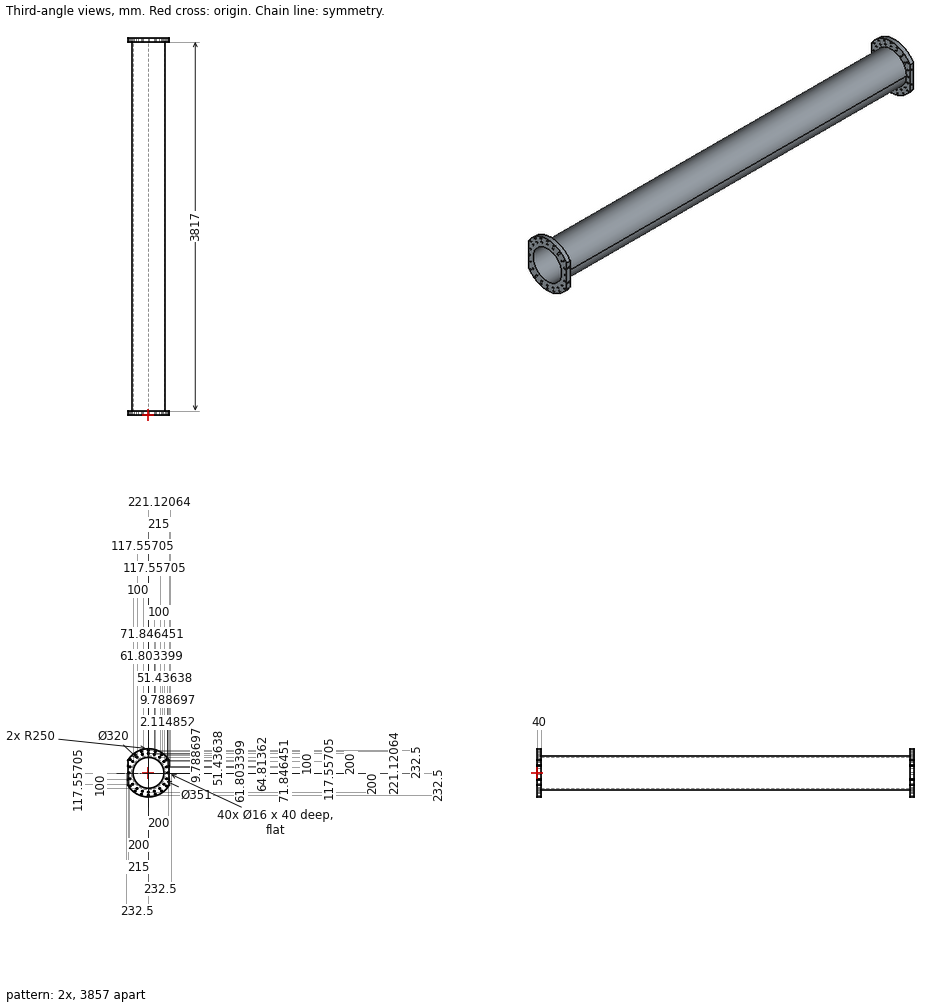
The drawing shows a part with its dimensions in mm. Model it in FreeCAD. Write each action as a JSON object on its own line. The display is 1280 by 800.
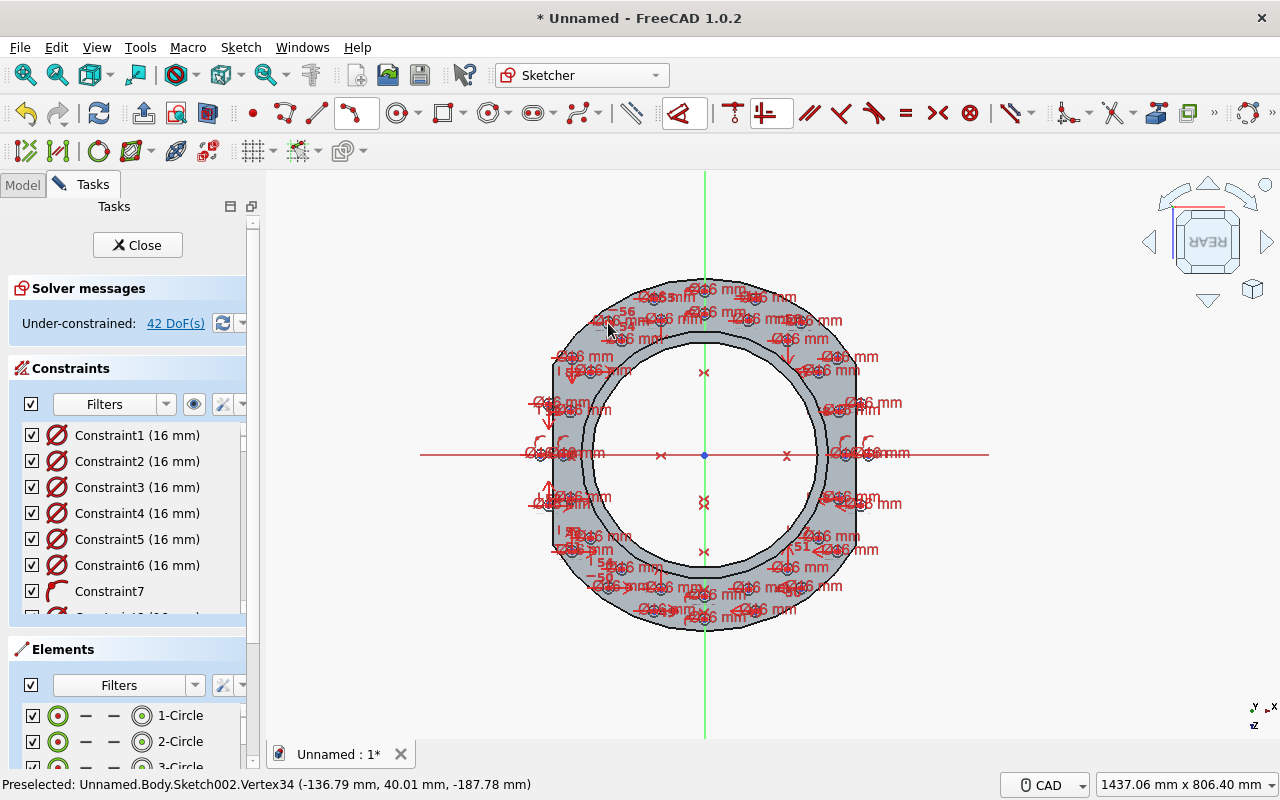
{"action": "left_click", "coordinate": [470, 455]}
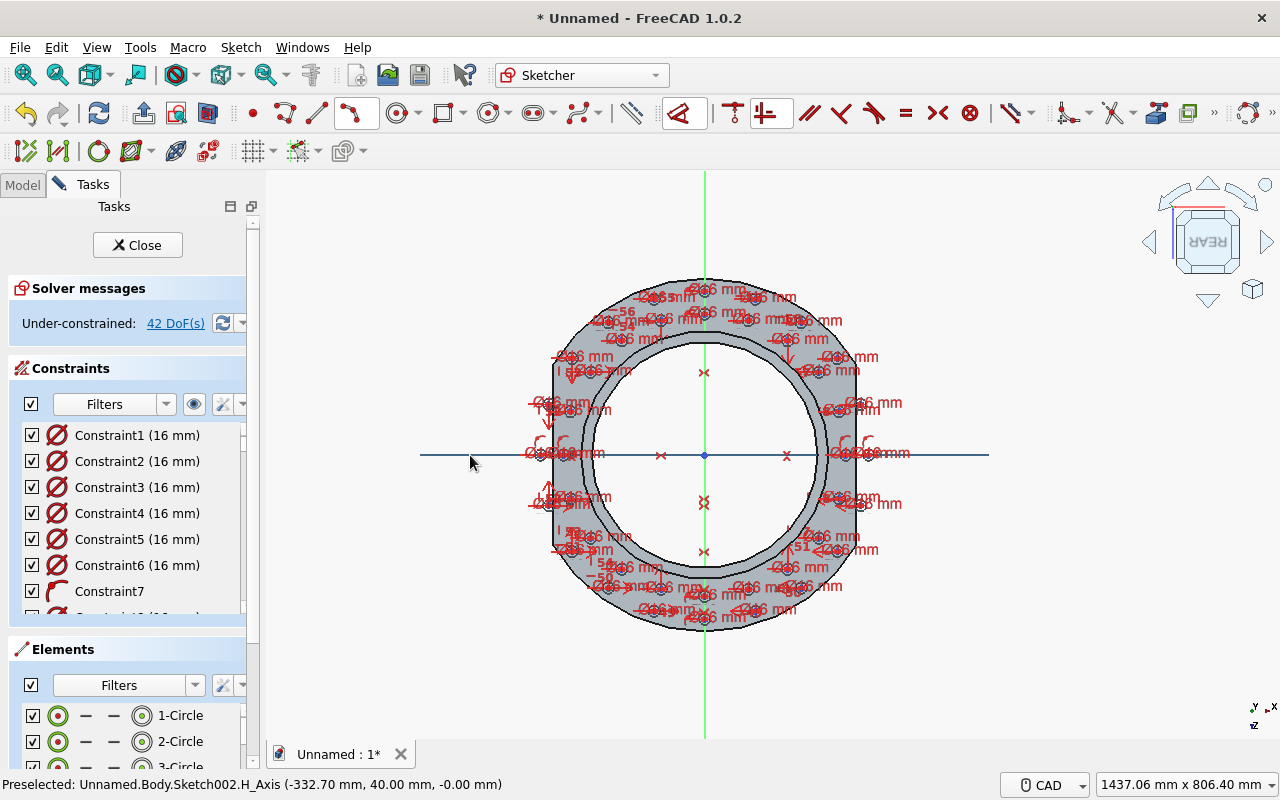
{"action": "key", "text": "s"}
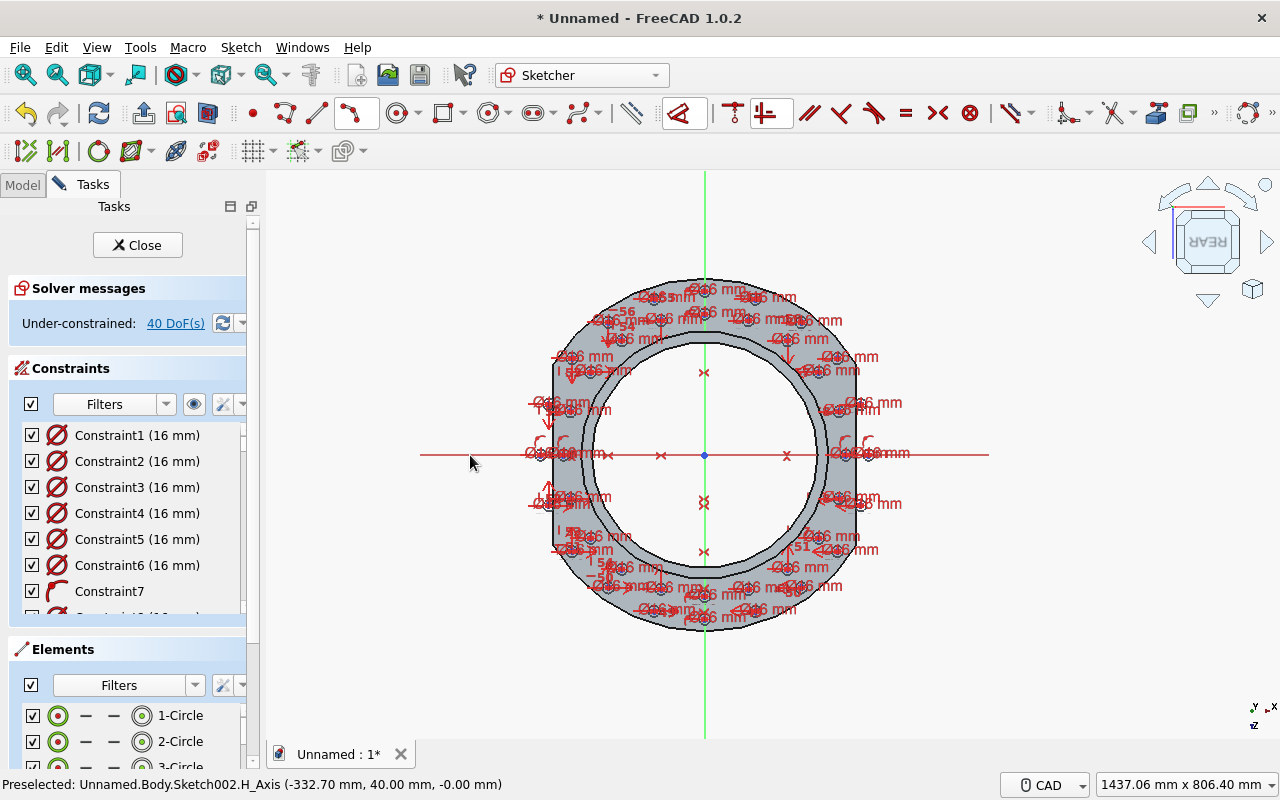
{"action": "scroll", "coordinate": [654, 611], "scroll_direction": "up", "scroll_amount": 4}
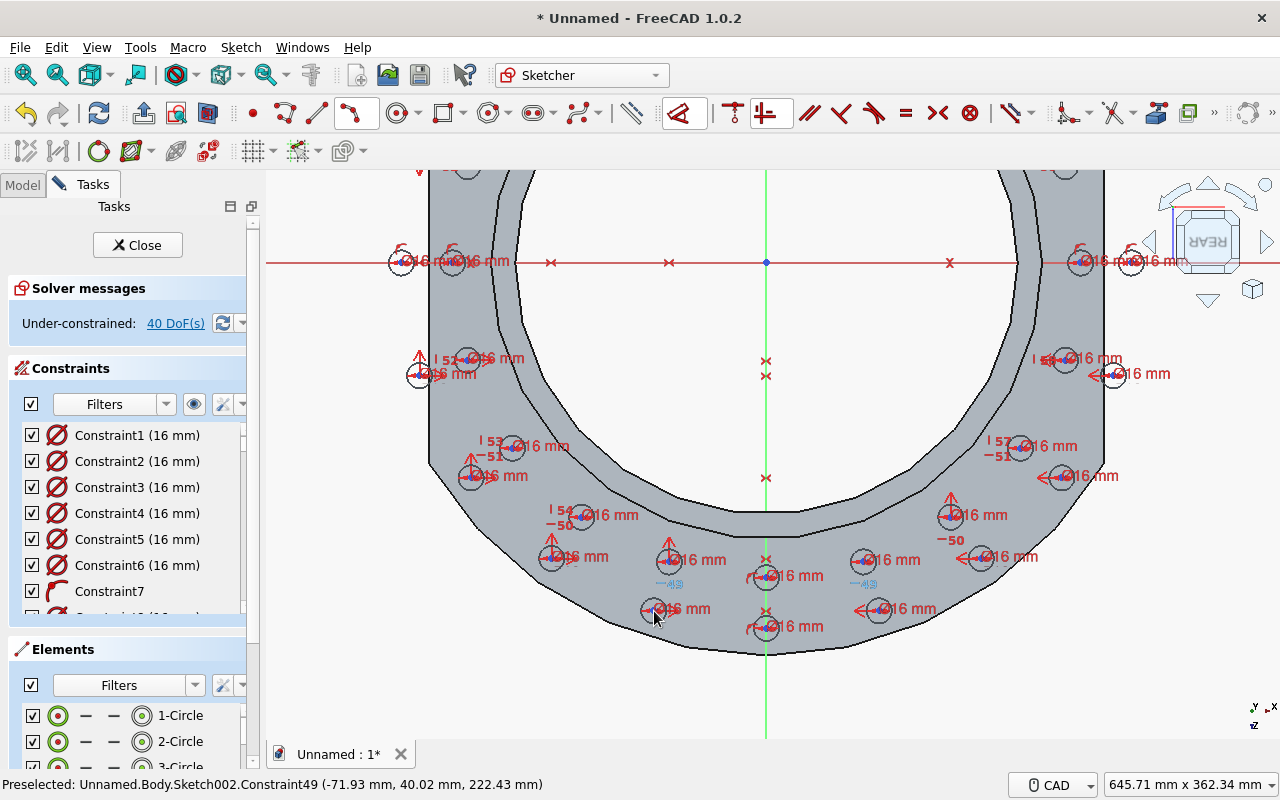
{"action": "left_click", "coordinate": [654, 611]}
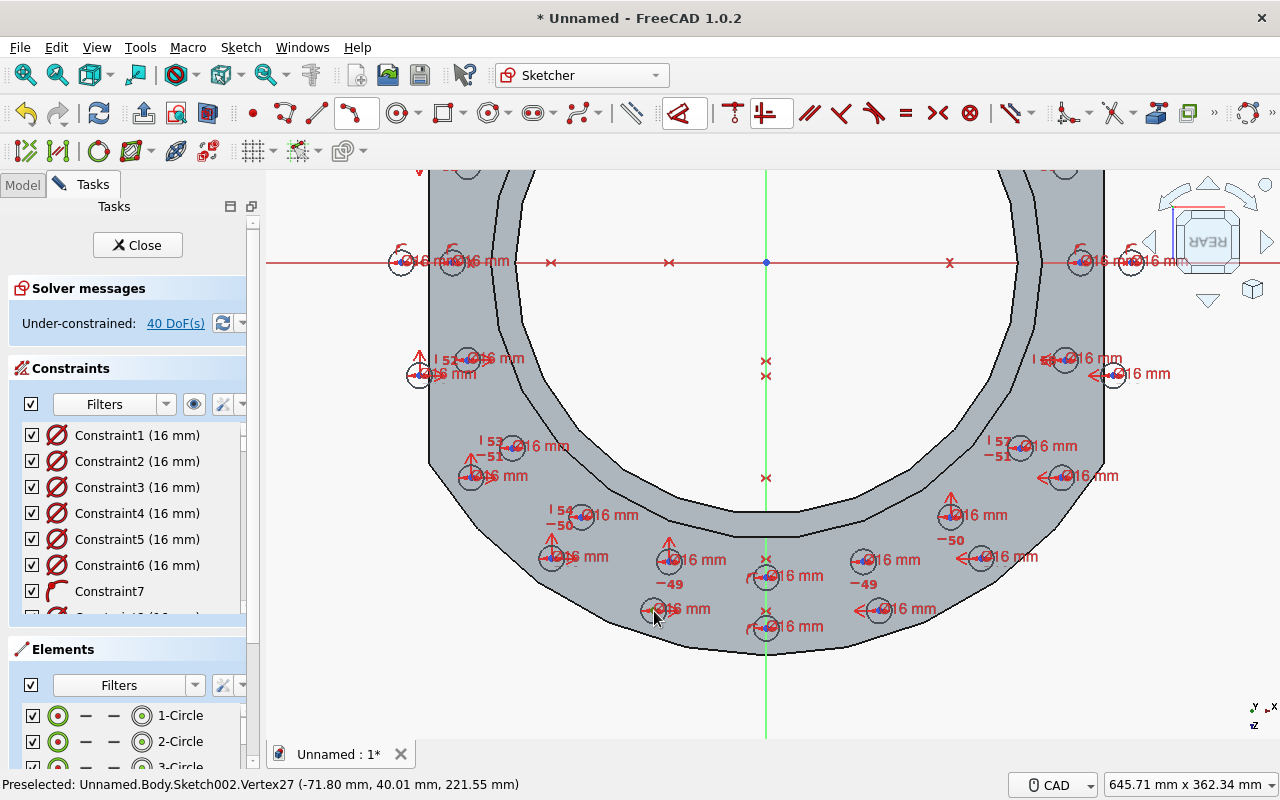
{"action": "scroll", "coordinate": [654, 611], "scroll_direction": "down", "scroll_amount": 4}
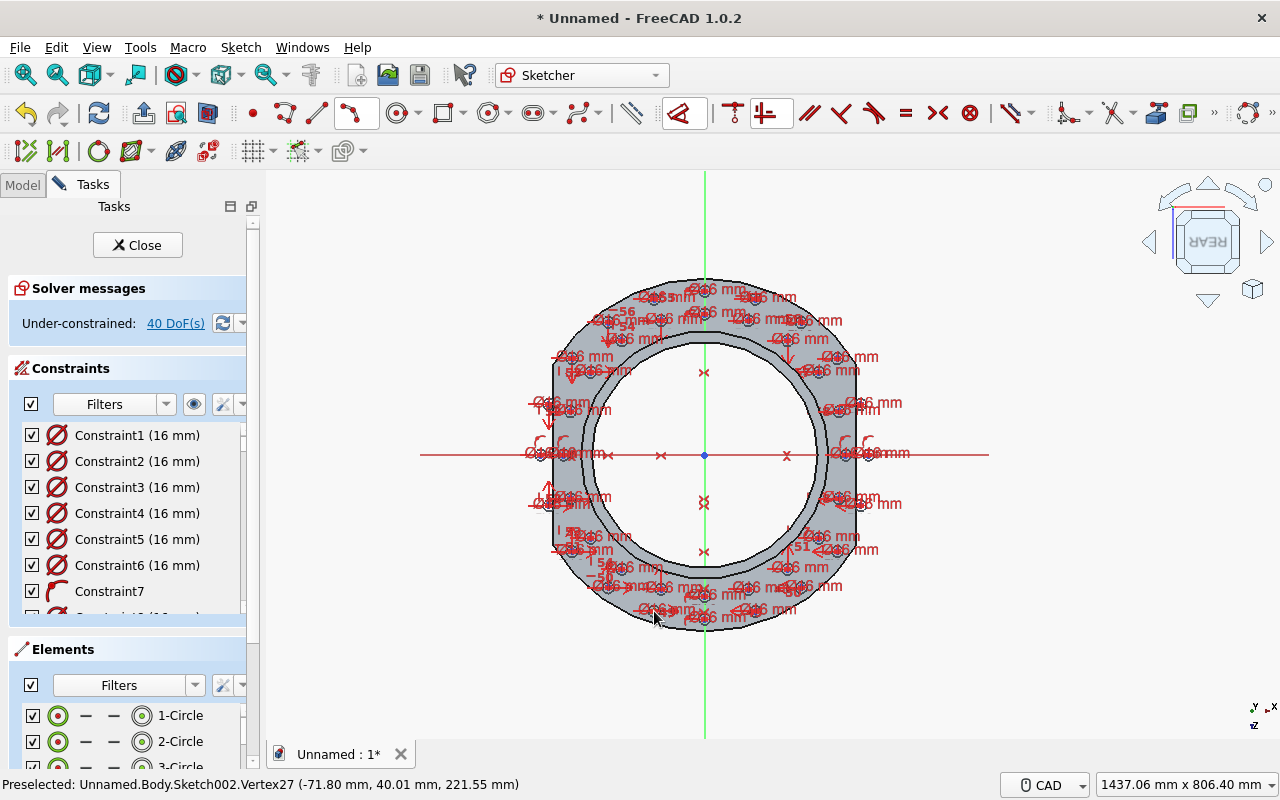
{"action": "left_click", "coordinate": [654, 299]}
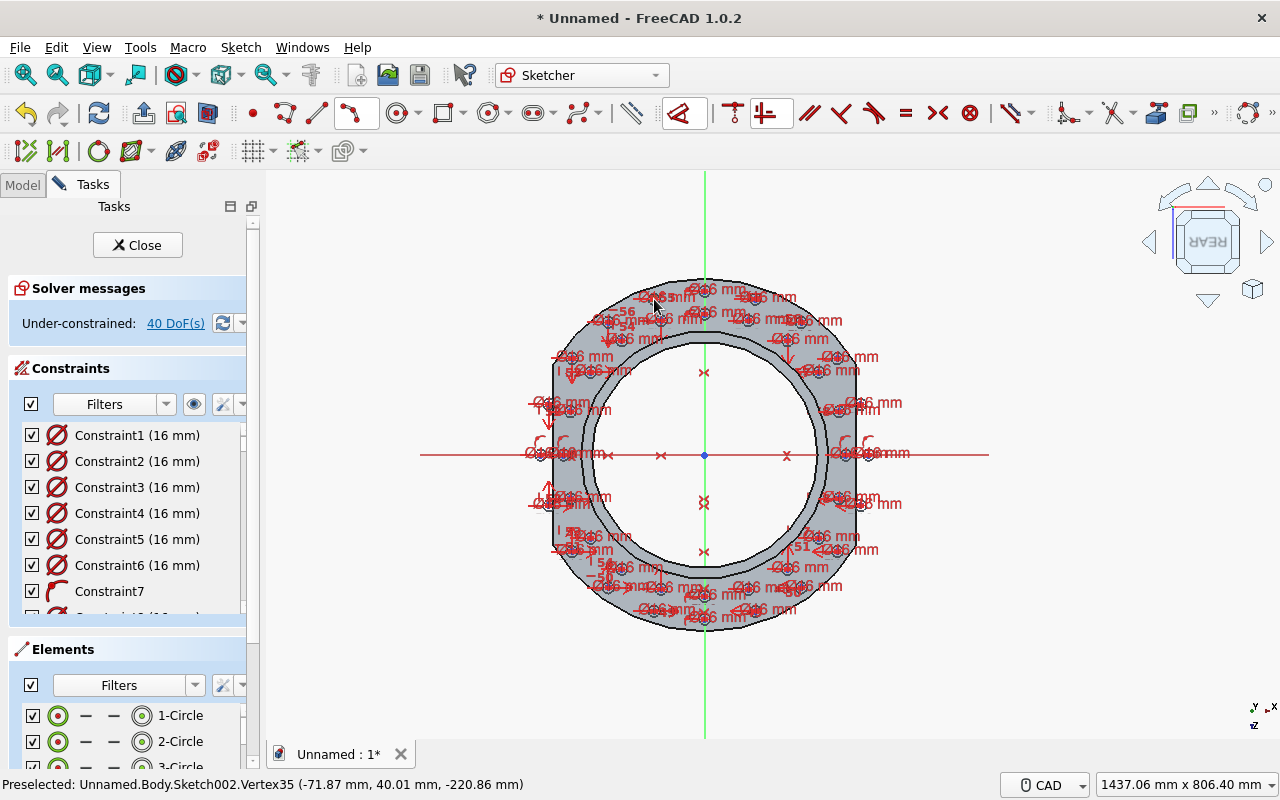
{"action": "left_click", "coordinate": [470, 455]}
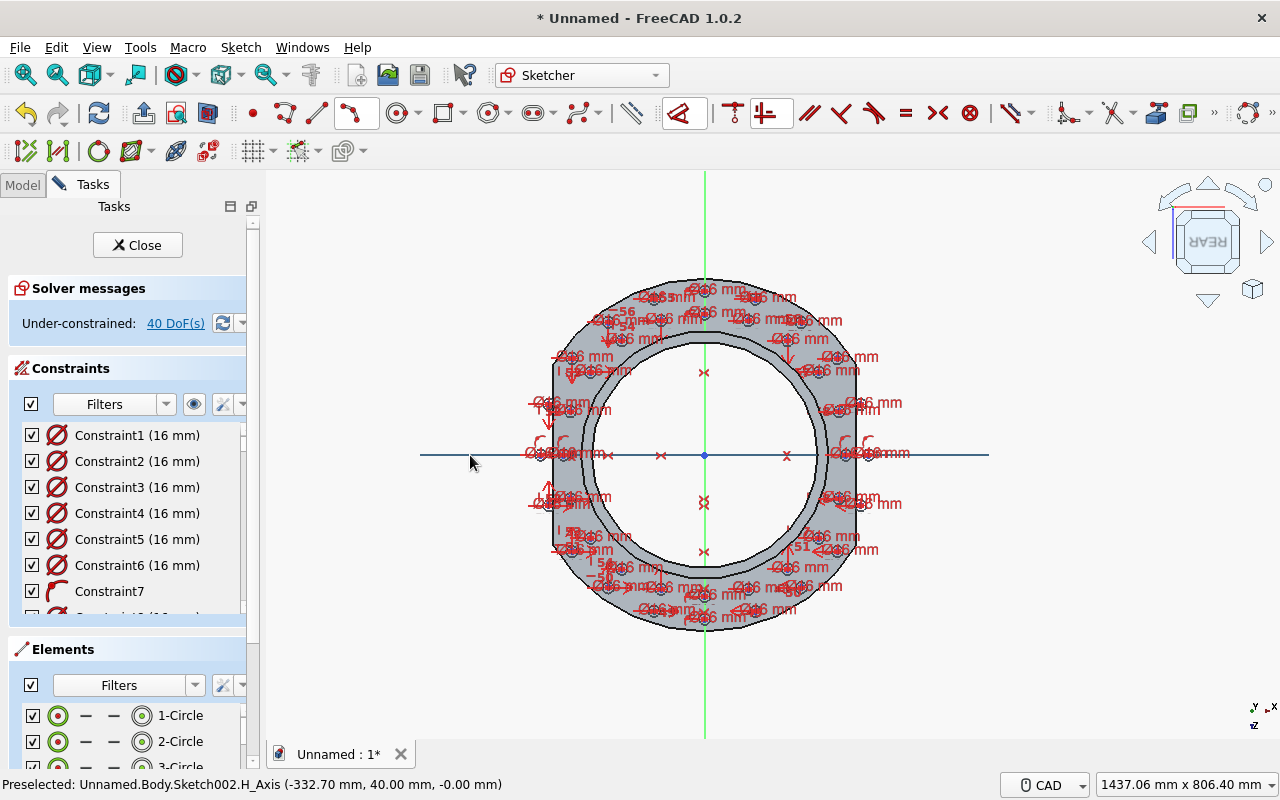
{"action": "left_click", "coordinate": [938, 114]}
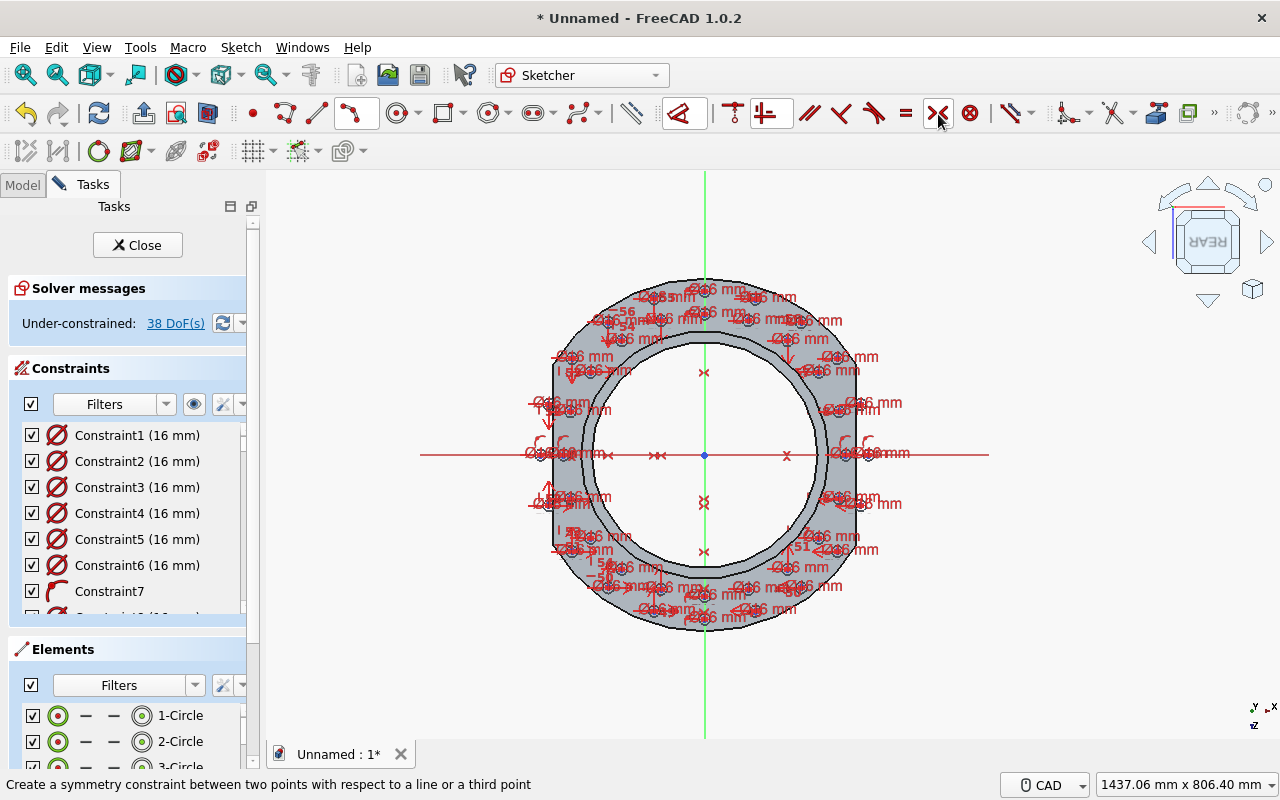
{"action": "left_click", "coordinate": [755, 611]}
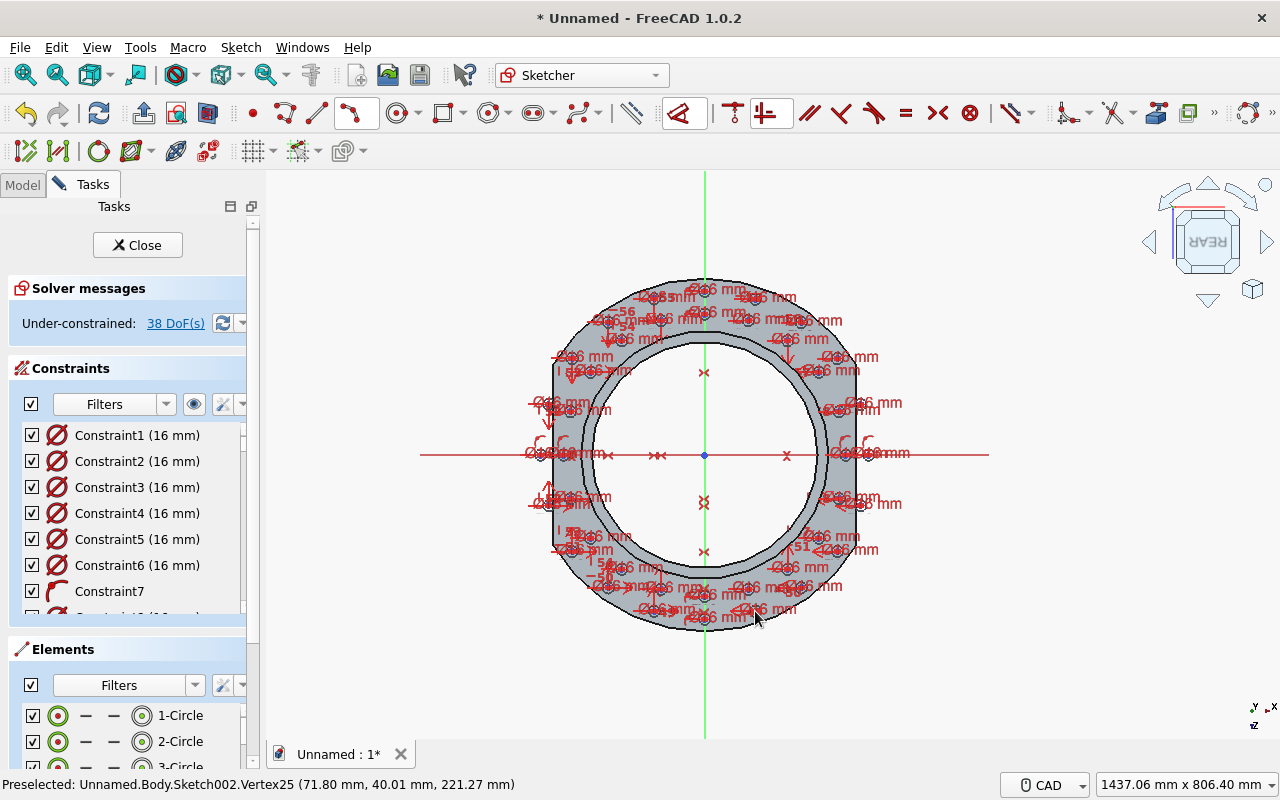
{"action": "scroll", "coordinate": [755, 299], "scroll_direction": "up", "scroll_amount": 4}